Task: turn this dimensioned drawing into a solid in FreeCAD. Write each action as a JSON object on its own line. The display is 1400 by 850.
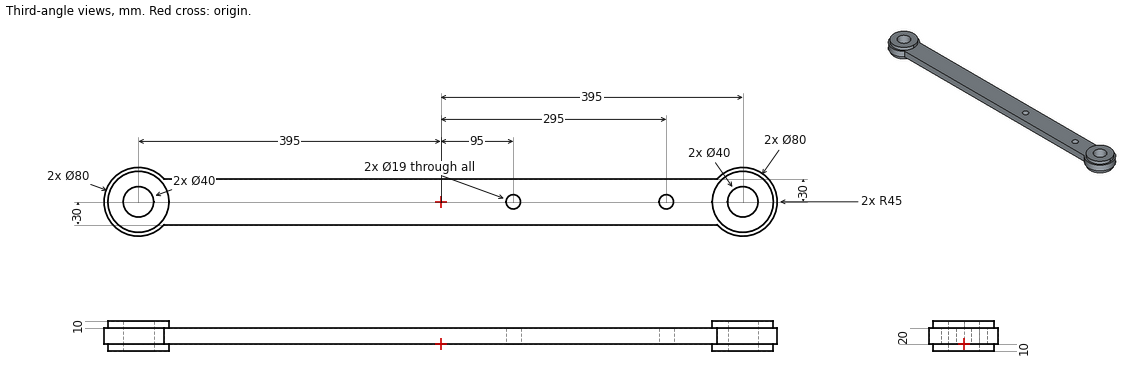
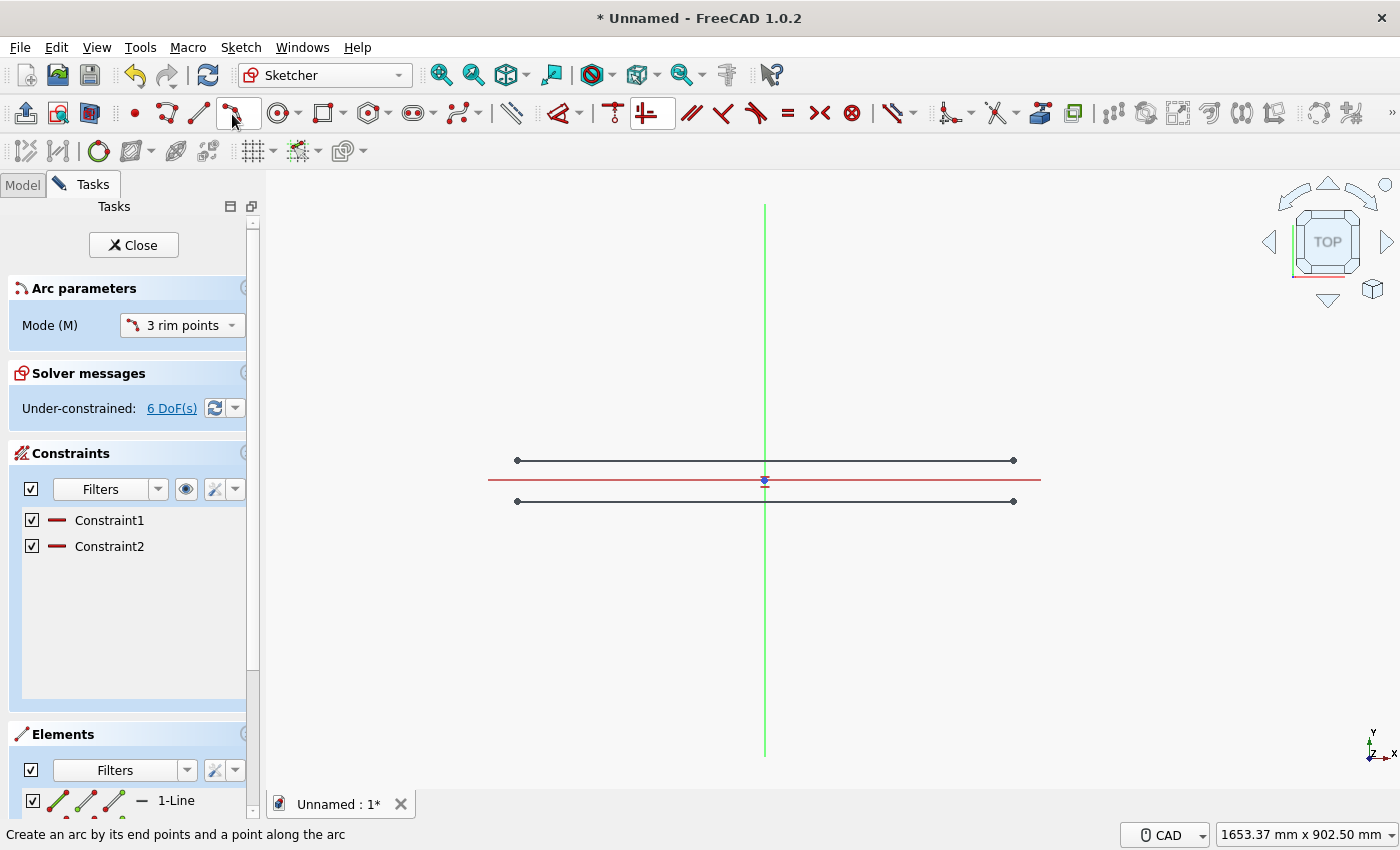
{"action": "left_click", "coordinate": [517, 461]}
{"action": "left_click", "coordinate": [517, 502]}
{"action": "left_click", "coordinate": [467, 466]}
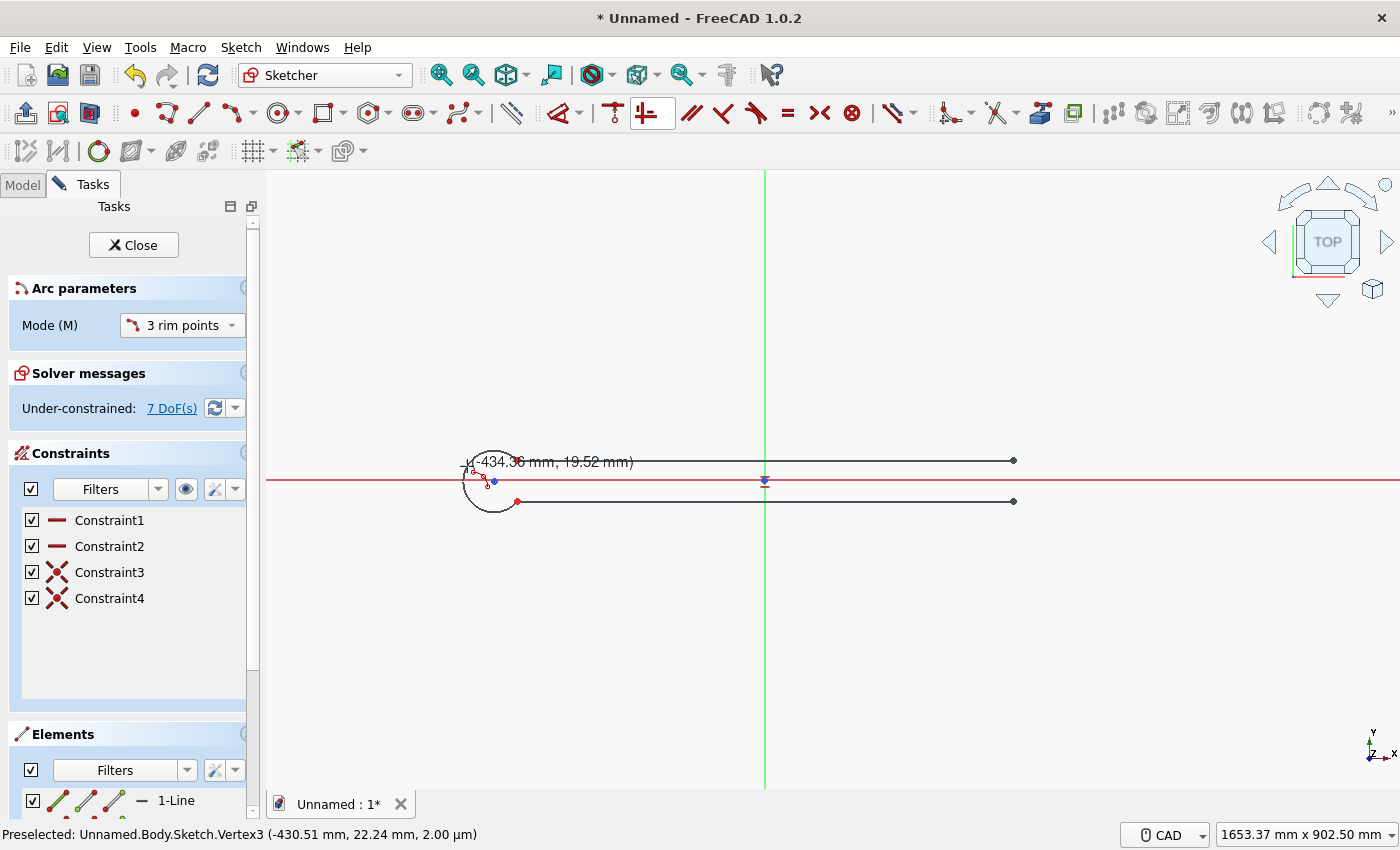
{"action": "left_click", "coordinate": [1013, 502]}
{"action": "left_click", "coordinate": [1013, 461]}
{"action": "left_click", "coordinate": [1063, 495]}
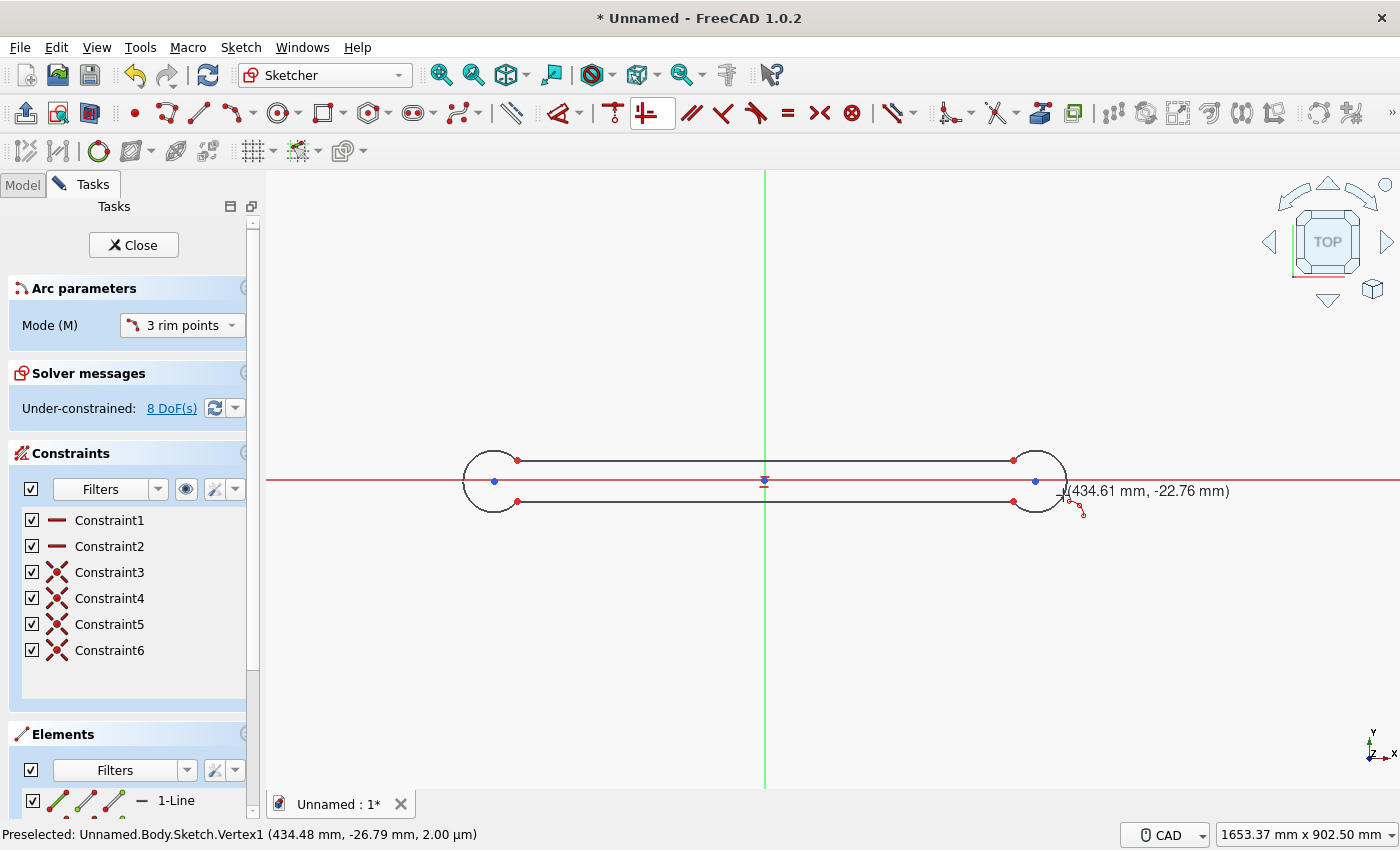
{"action": "left_click", "coordinate": [278, 114]}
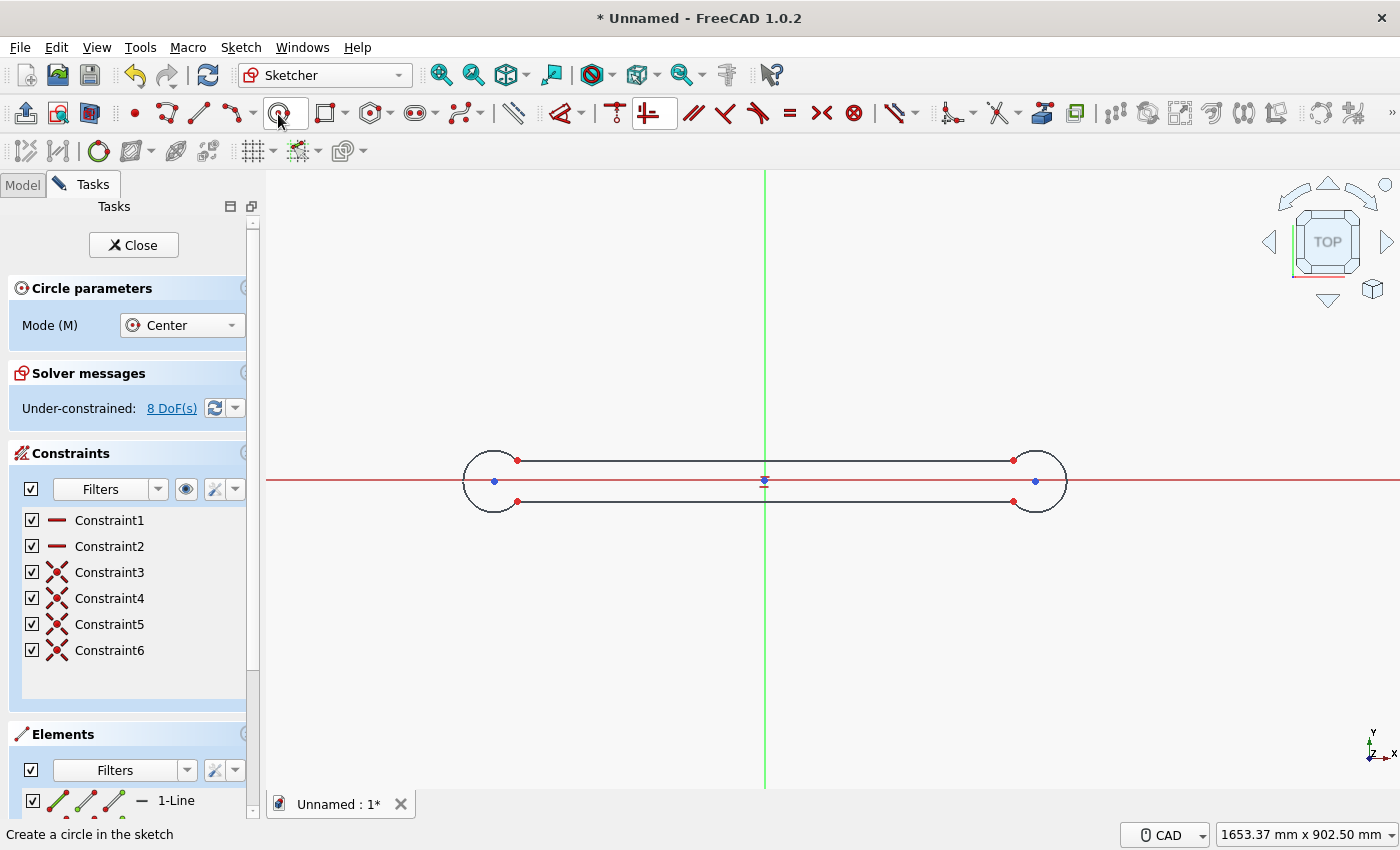
{"action": "scroll", "coordinate": [494, 480], "scroll_direction": "up", "scroll_amount": 3}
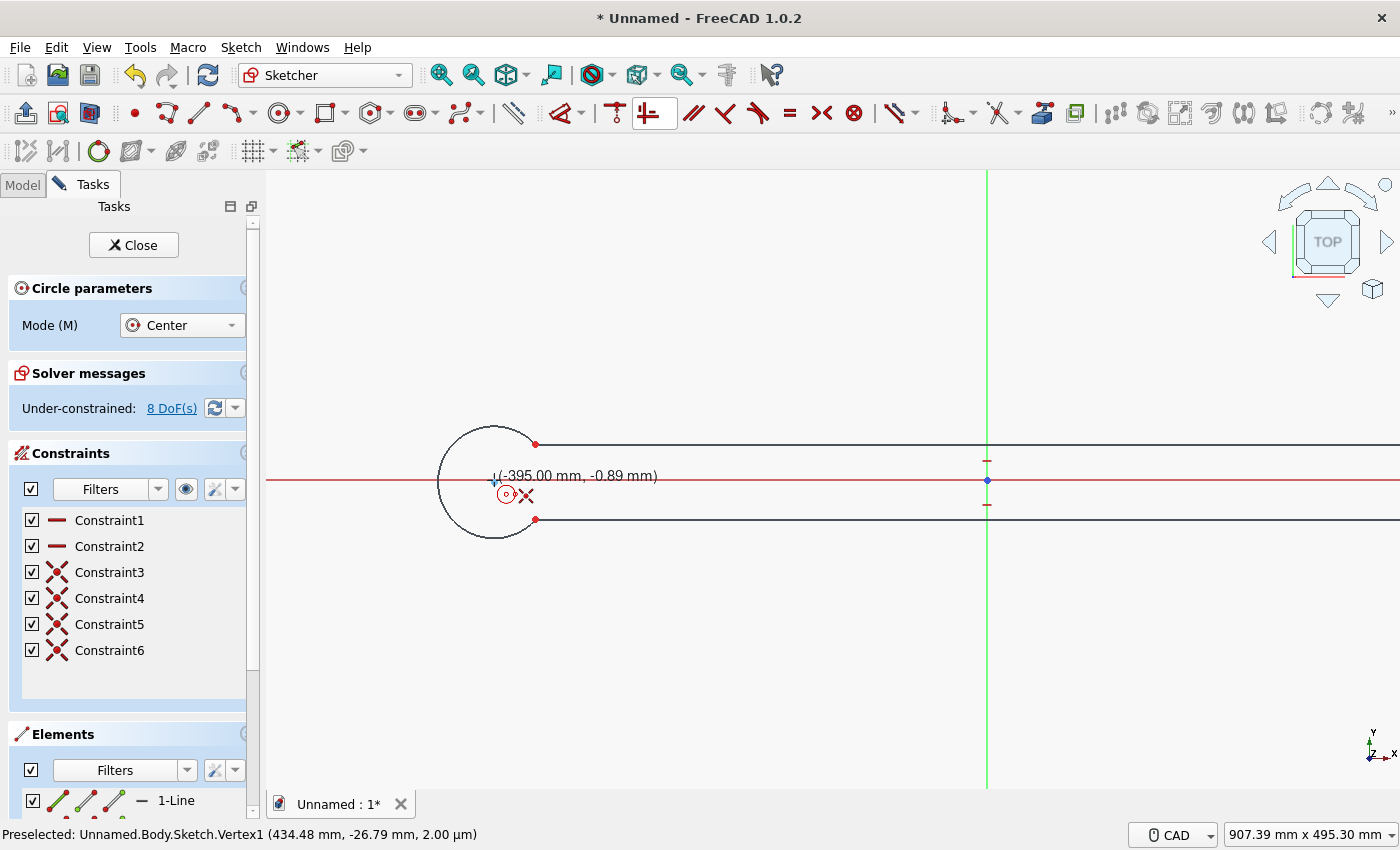
{"action": "left_click", "coordinate": [494, 480]}
{"action": "left_click", "coordinate": [512, 463]}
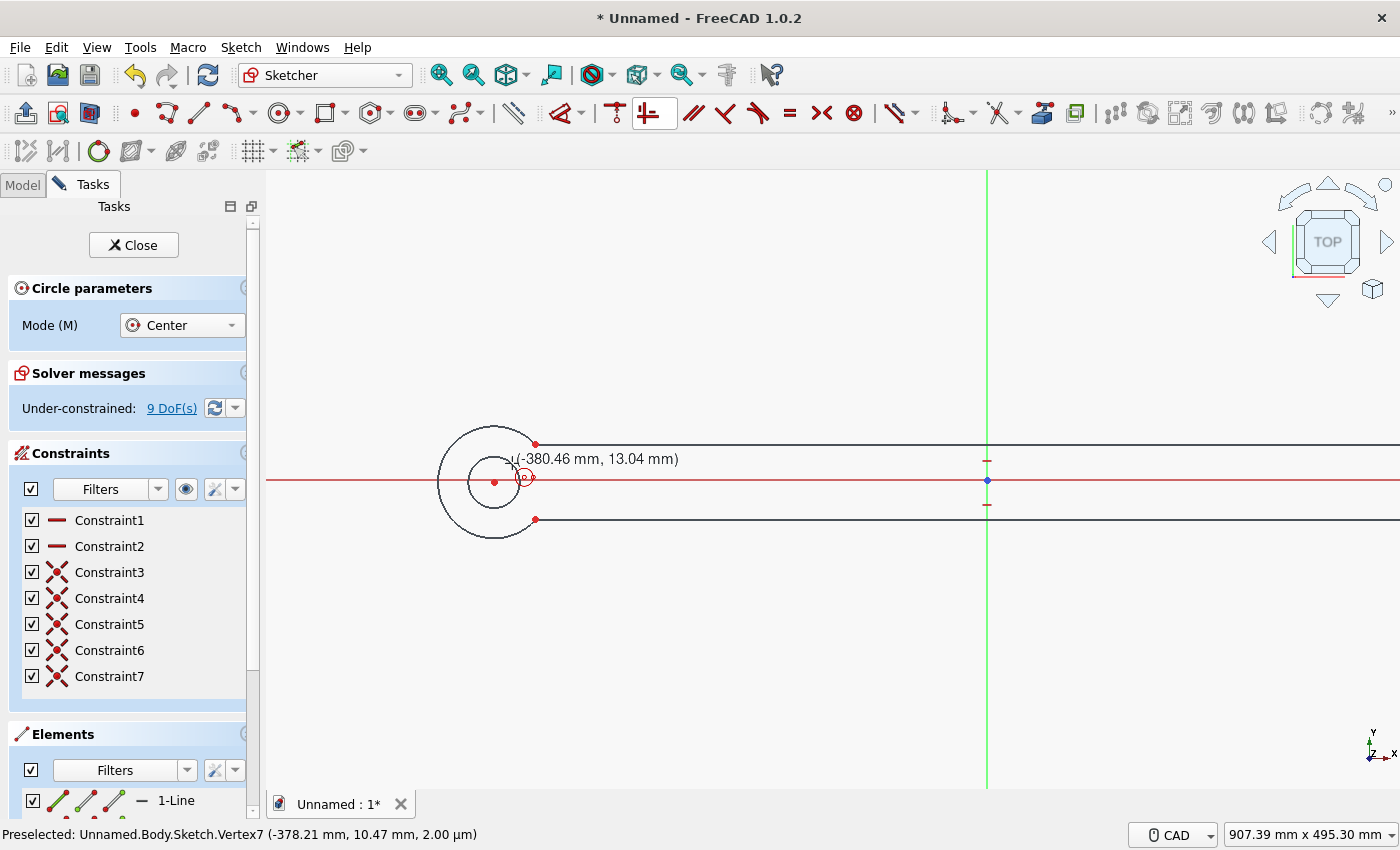
{"action": "scroll", "coordinate": [493, 479], "scroll_direction": "down", "scroll_amount": 3}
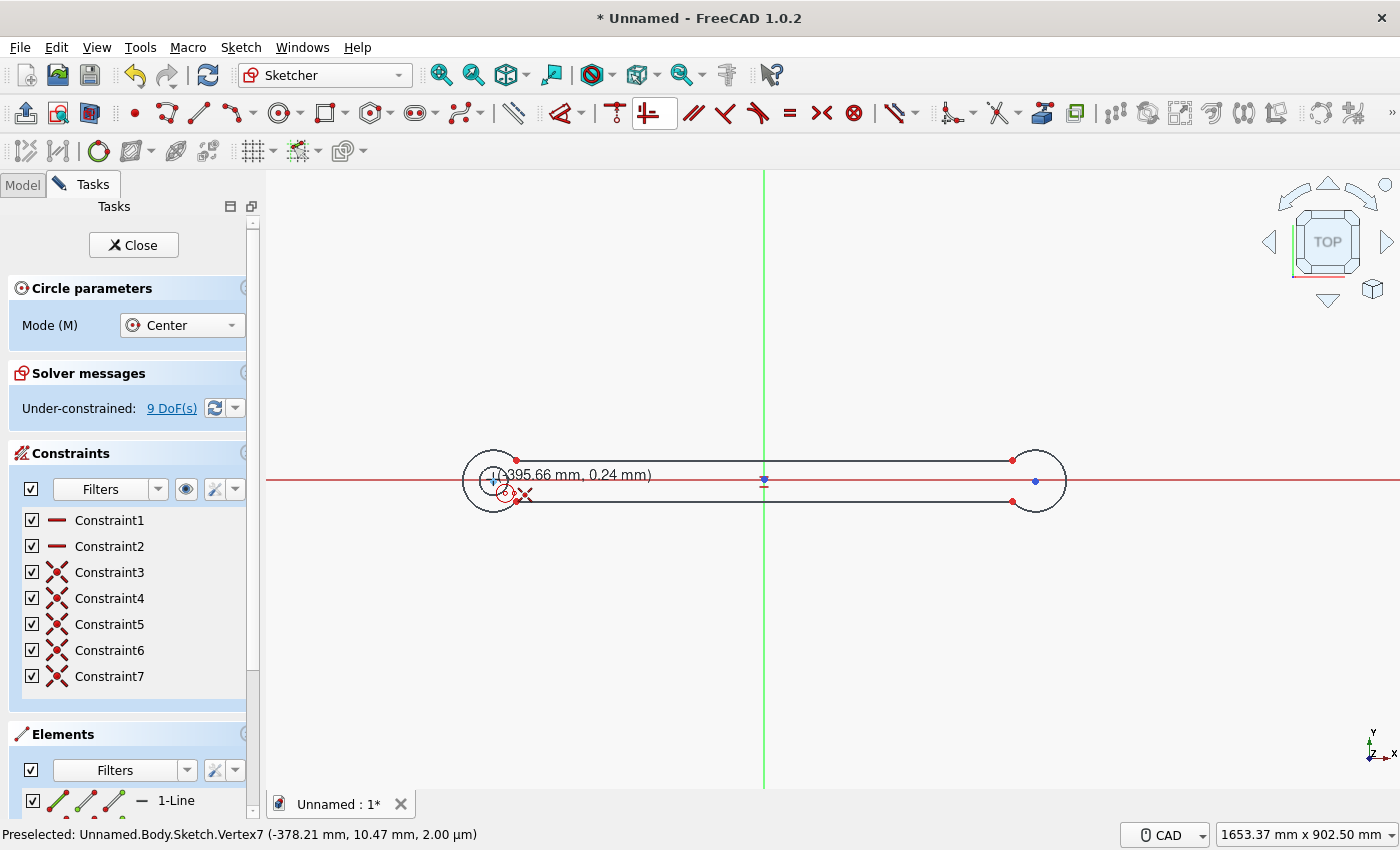
{"action": "scroll", "coordinate": [1035, 480], "scroll_direction": "up", "scroll_amount": 3}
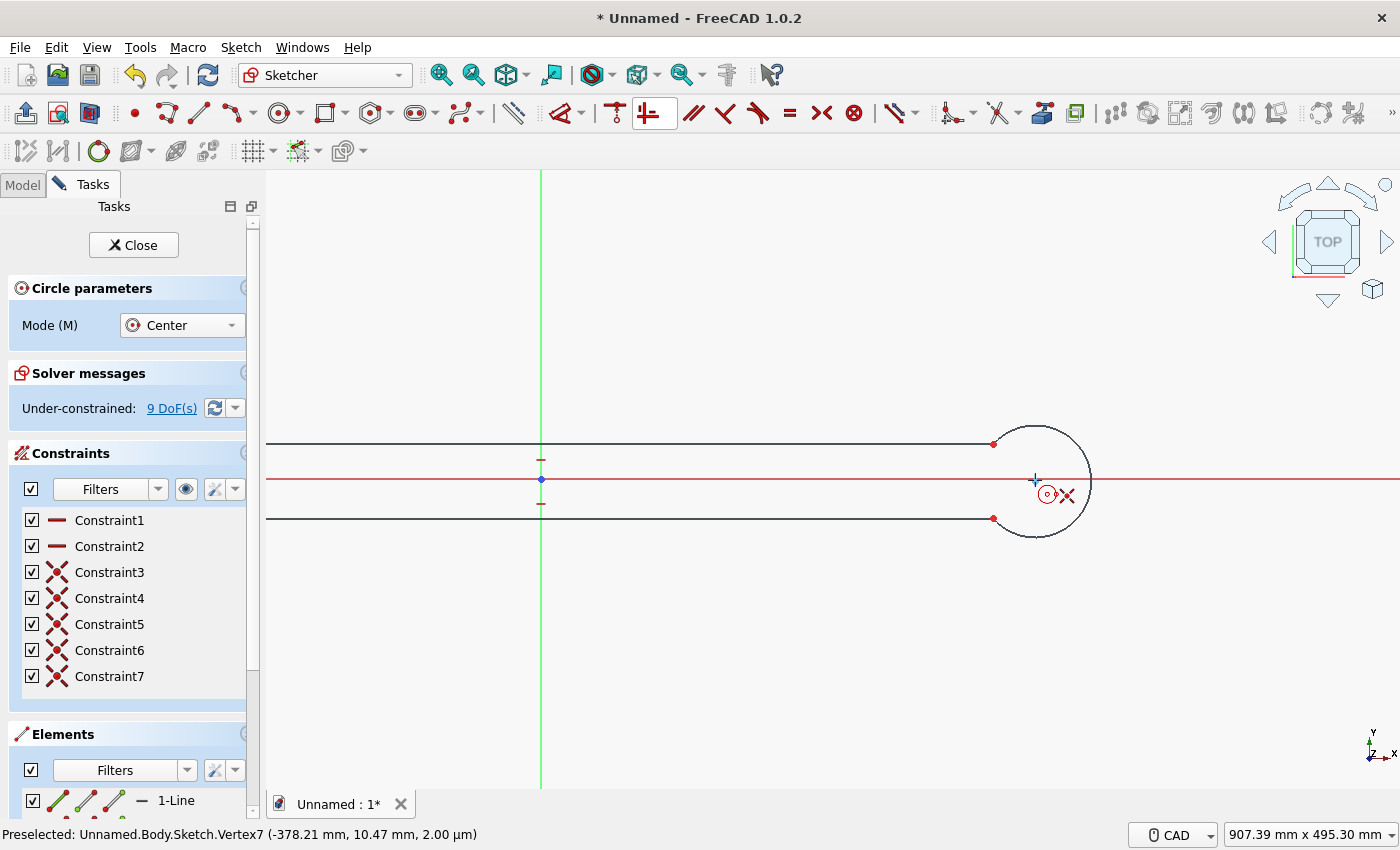
{"action": "left_click", "coordinate": [1035, 479]}
{"action": "left_click", "coordinate": [1053, 462]}
{"action": "key", "text": "Escape"}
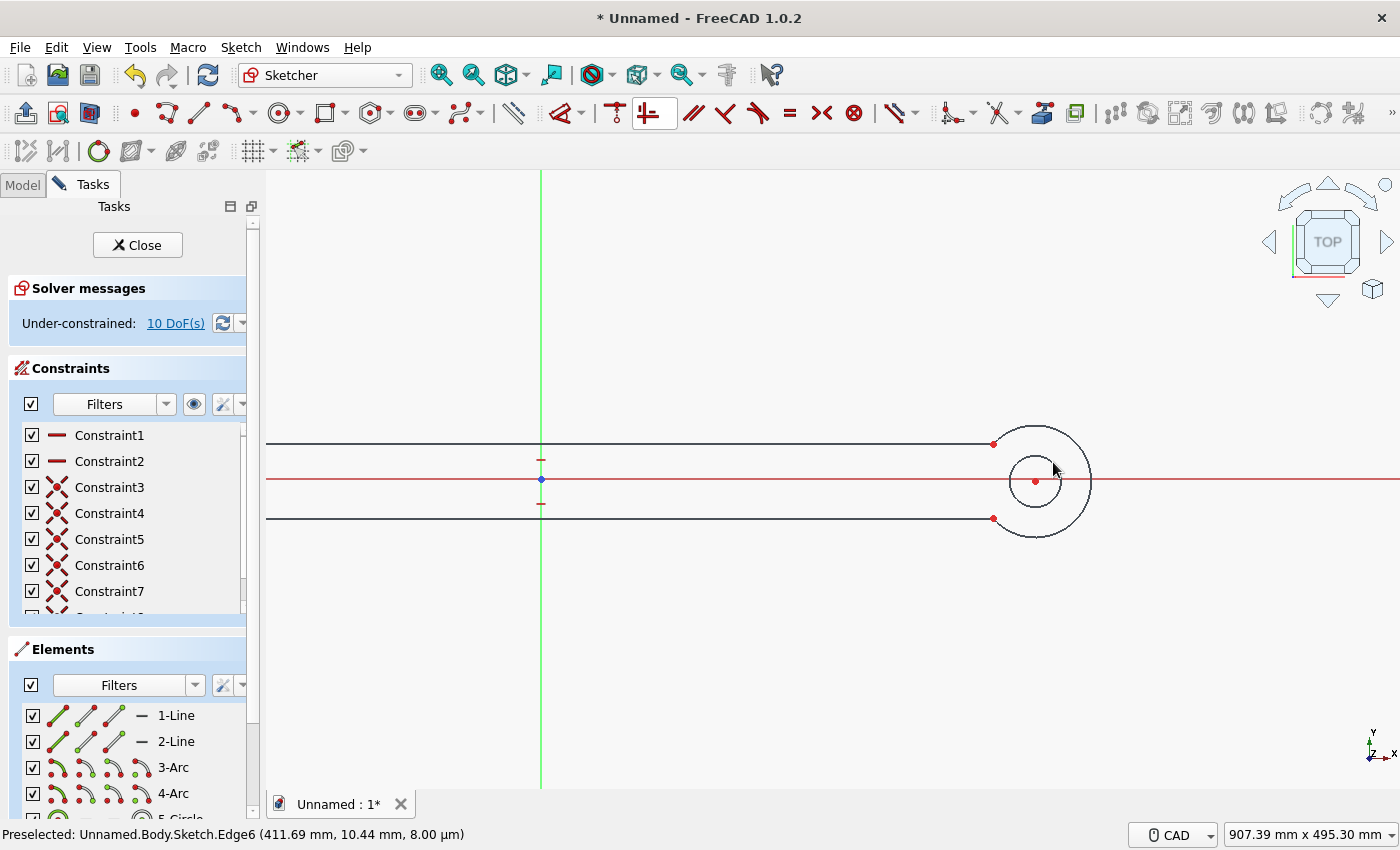
{"action": "scroll", "coordinate": [1036, 480], "scroll_direction": "down", "scroll_amount": 3}